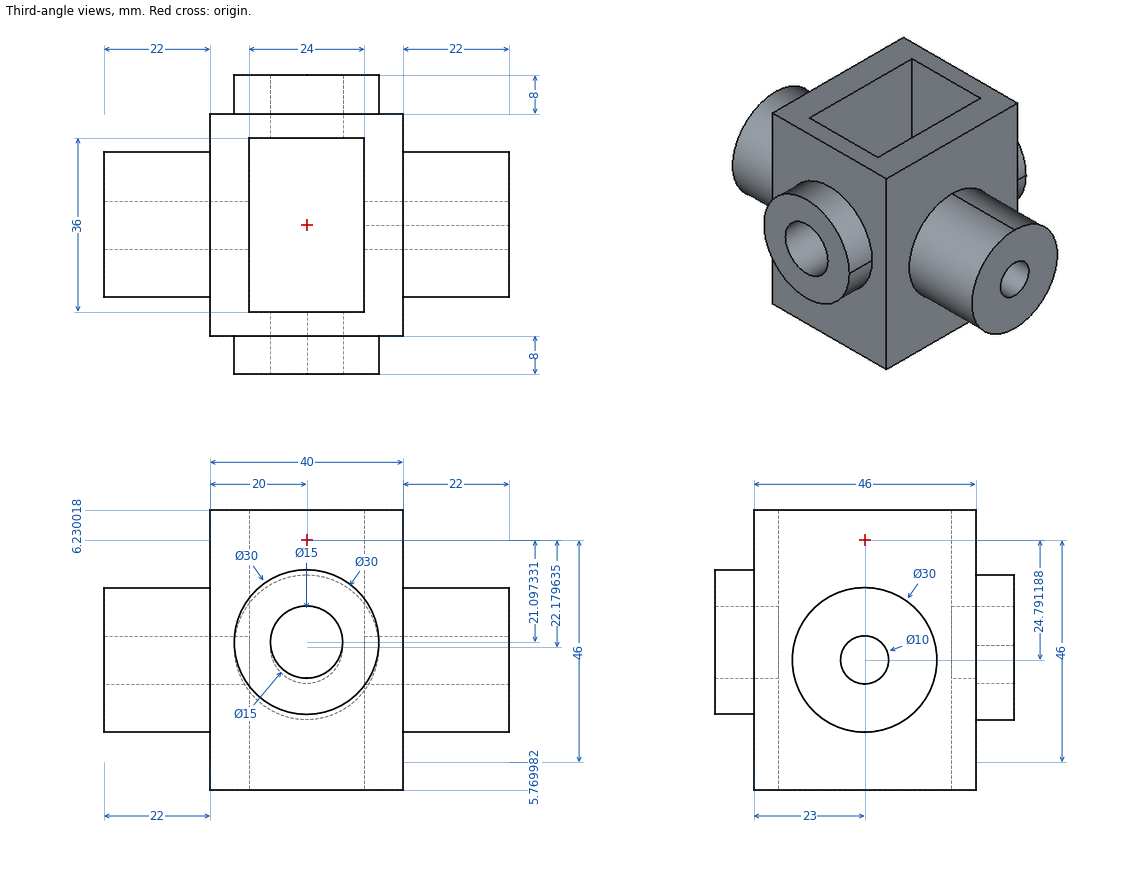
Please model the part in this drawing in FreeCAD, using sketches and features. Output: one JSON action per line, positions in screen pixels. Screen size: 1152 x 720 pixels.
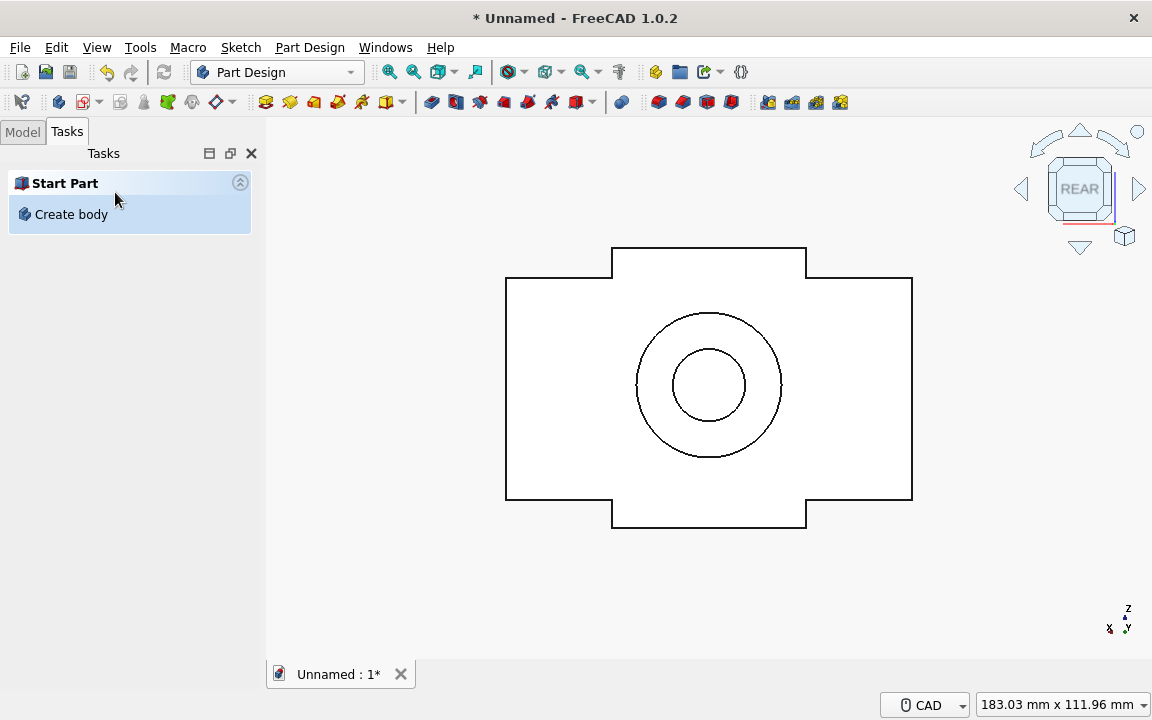
{"action": "key", "text": "0"}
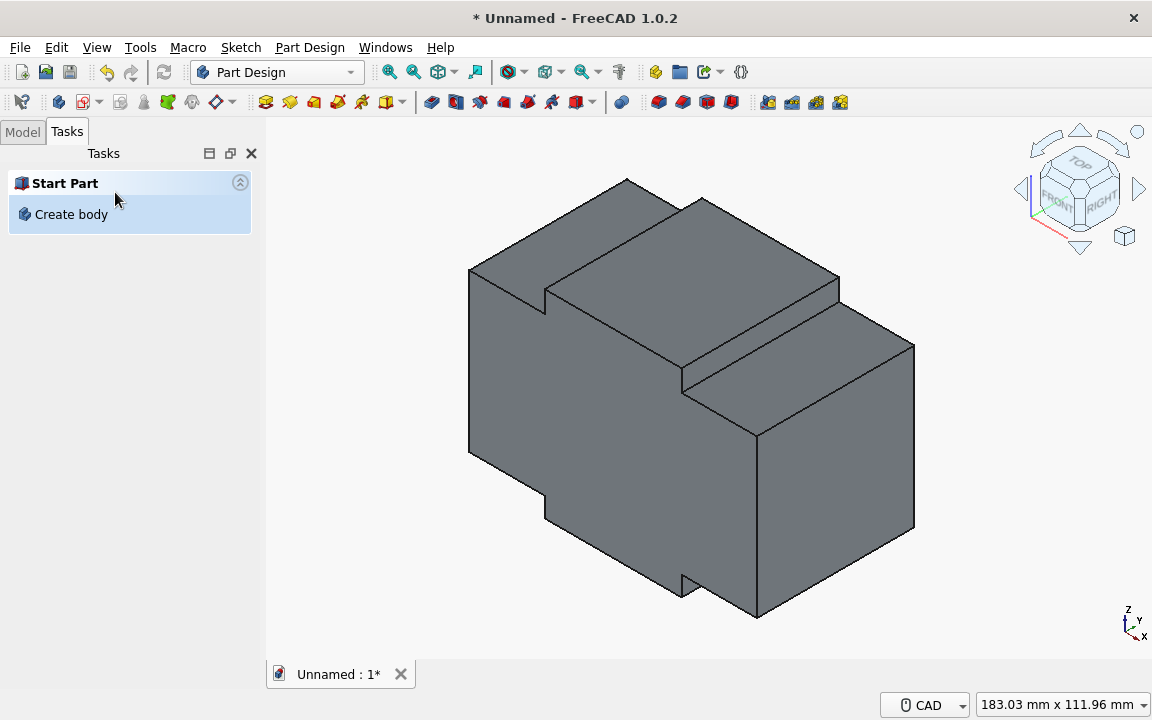
{"action": "left_click", "coordinate": [692, 282]}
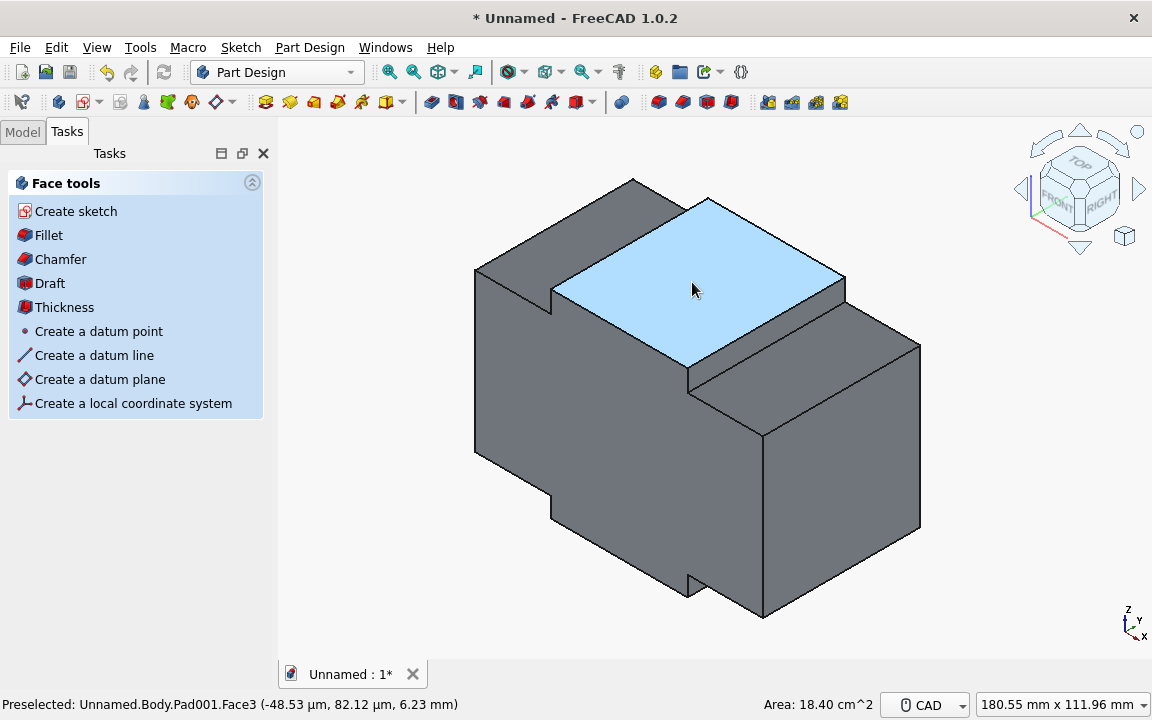
{"action": "left_click", "coordinate": [84, 102]}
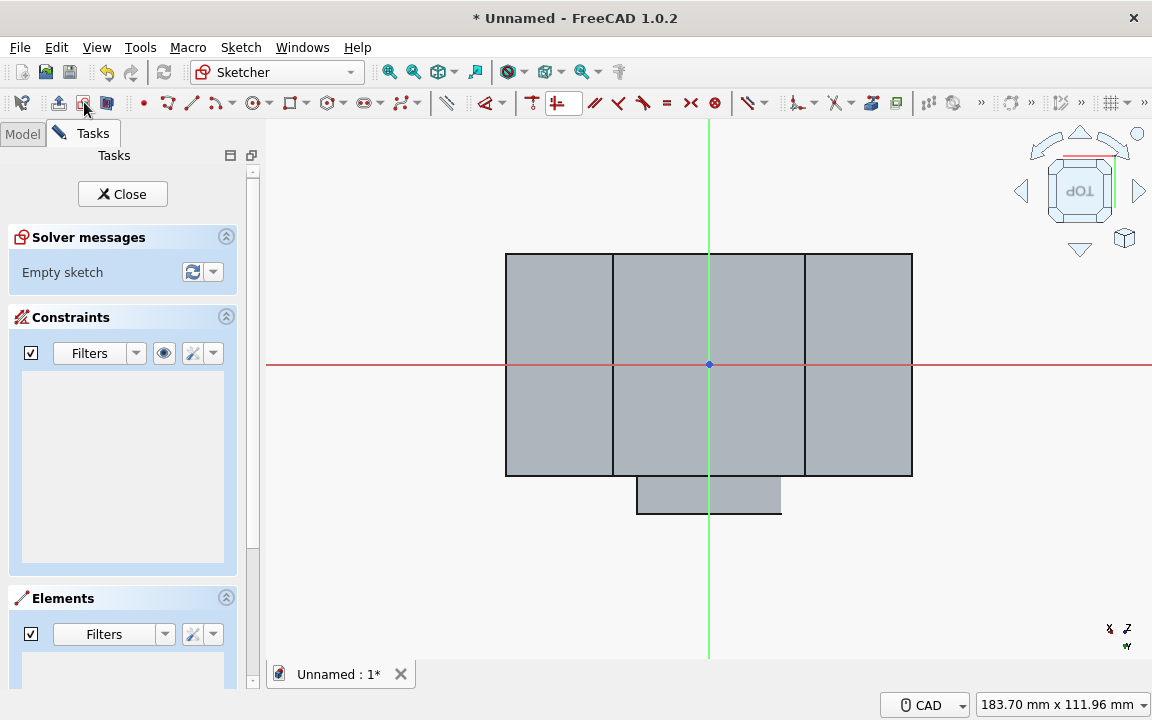
{"action": "scroll", "coordinate": [792, 336], "scroll_direction": "up", "scroll_amount": 3}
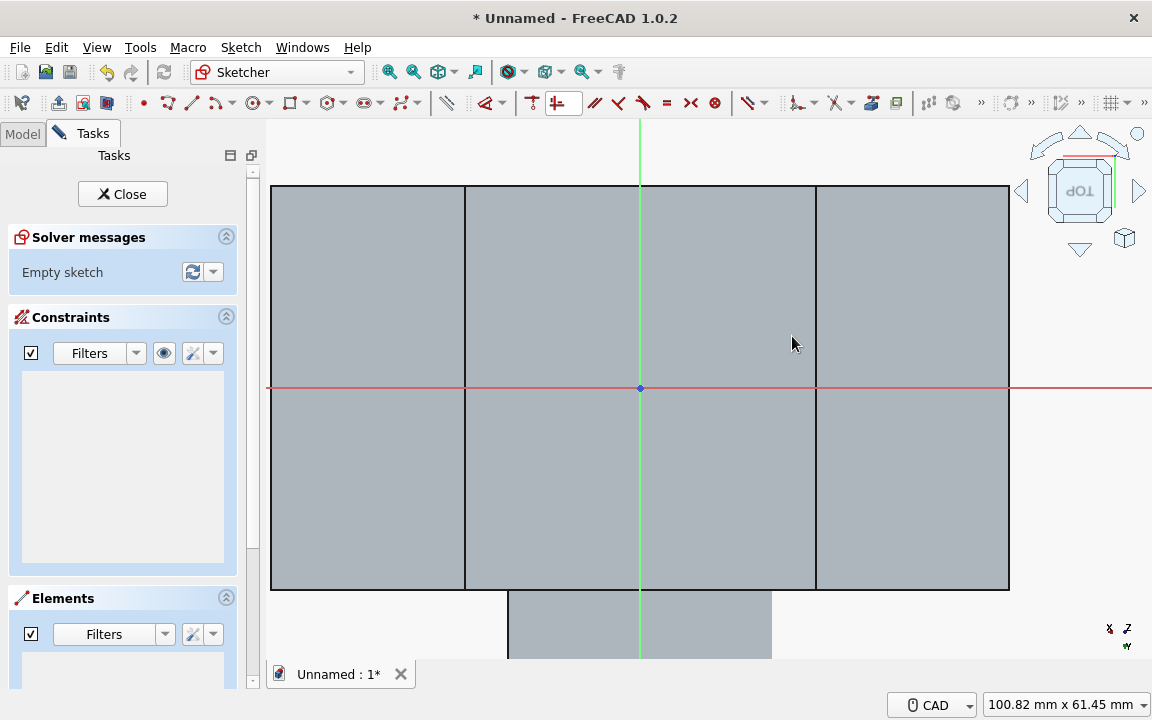
{"action": "key", "text": "g v"}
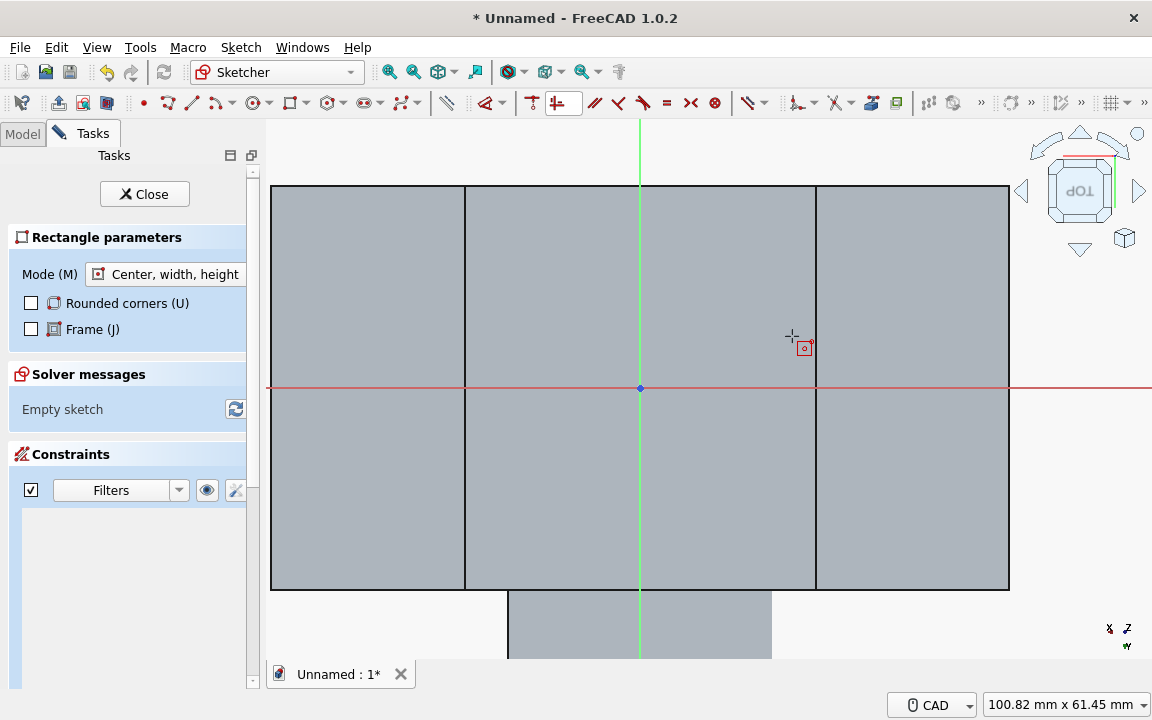
{"action": "left_click", "coordinate": [640, 388]}
{"action": "left_click", "coordinate": [746, 230]}
{"action": "key", "text": "Escape"}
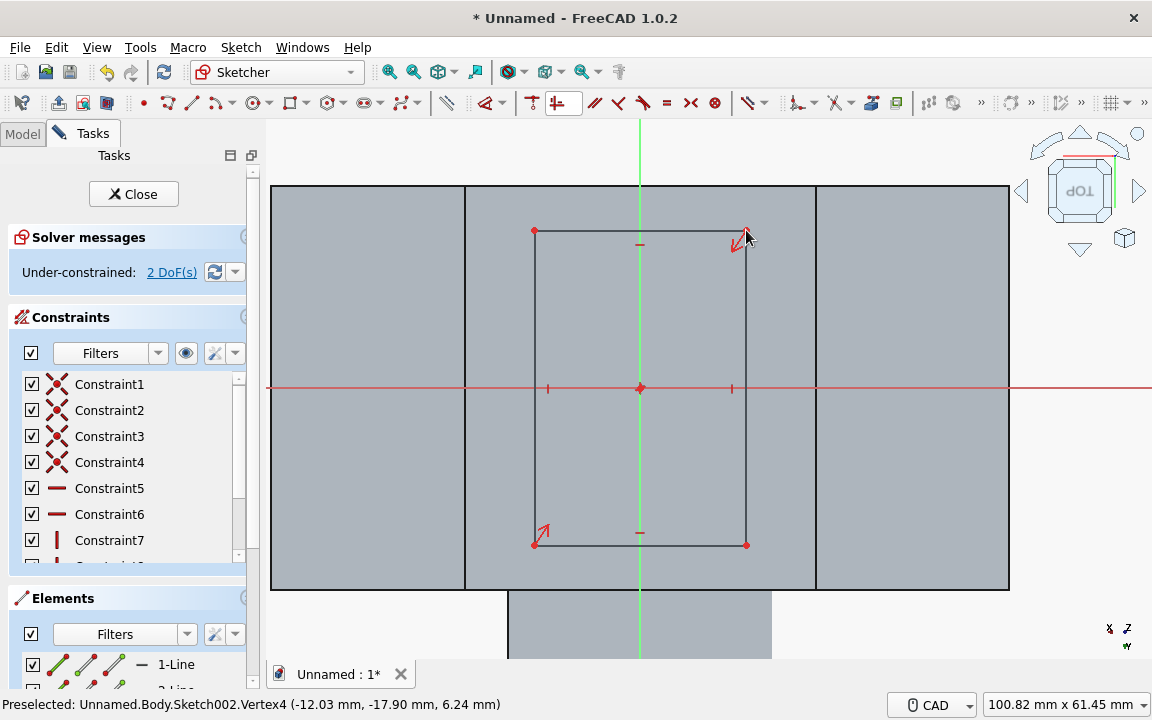
{"action": "left_click", "coordinate": [486, 104]}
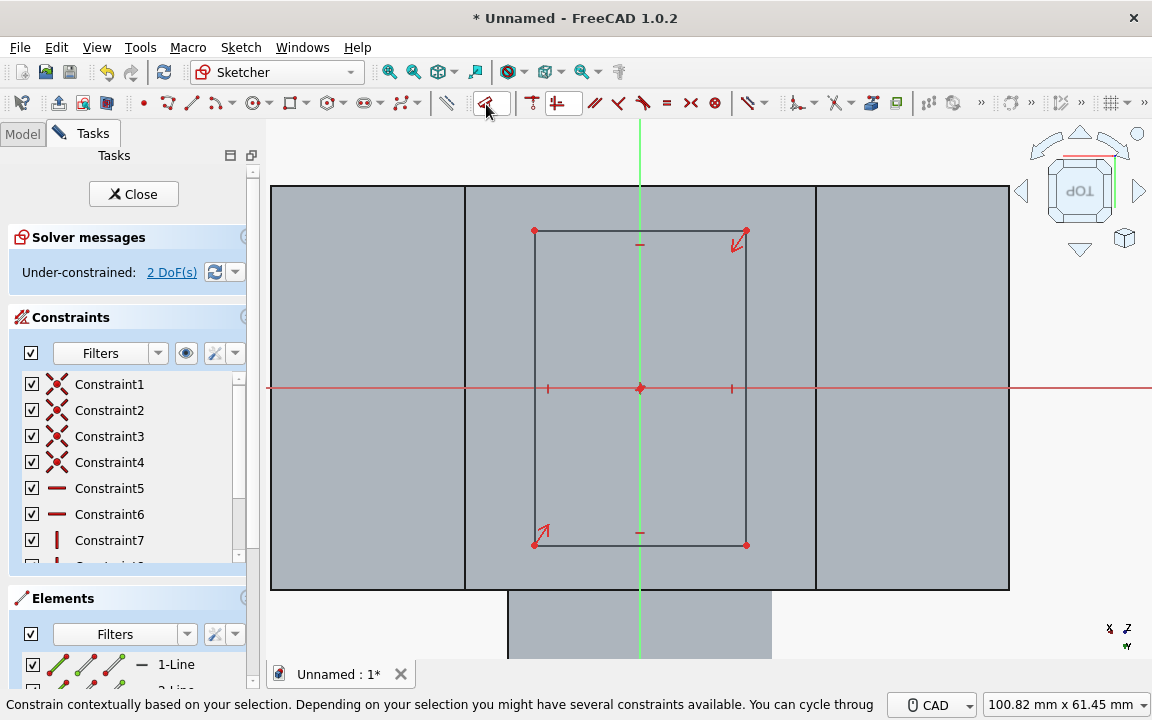
{"action": "left_click", "coordinate": [598, 546]}
{"action": "left_click", "coordinate": [592, 580]}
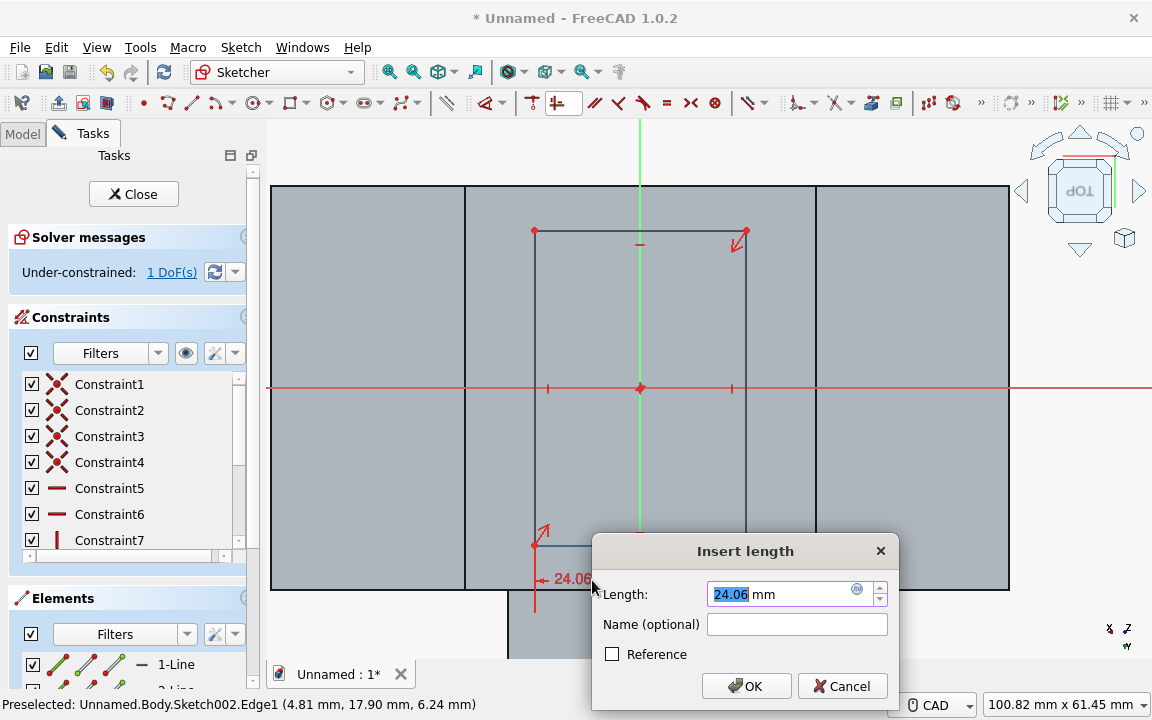
{"action": "type", "text": "24"}
{"action": "key", "text": "Return"}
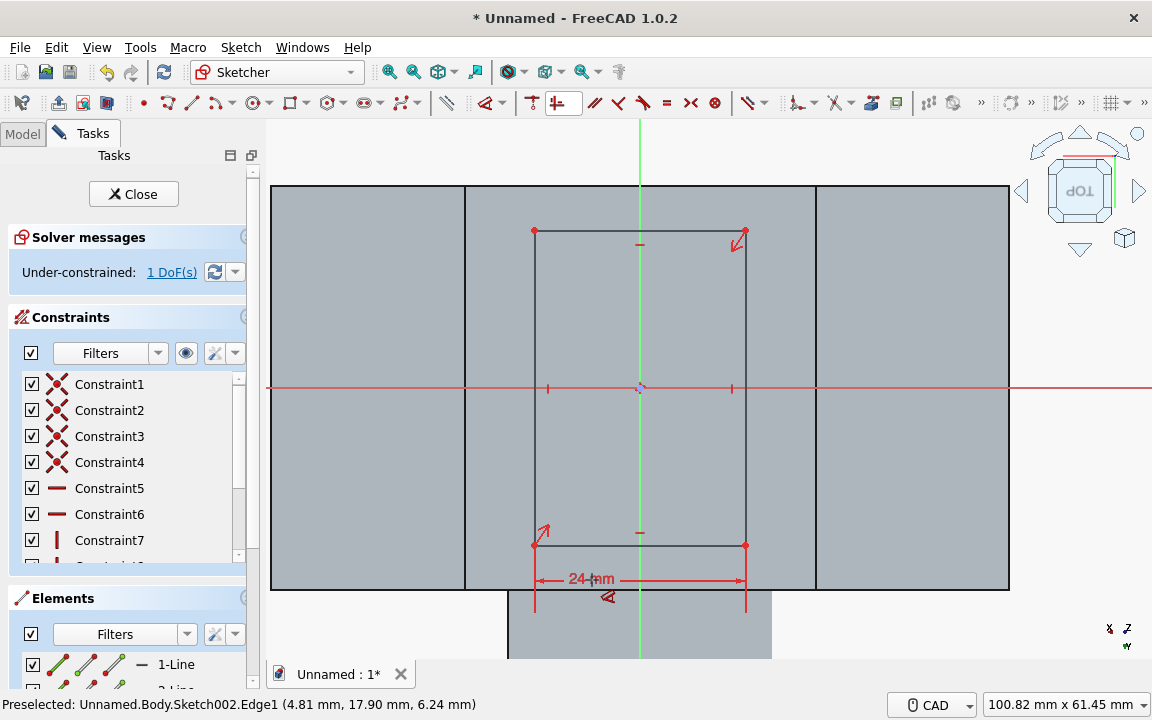
{"action": "left_click", "coordinate": [746, 451]}
{"action": "left_click", "coordinate": [780, 316]}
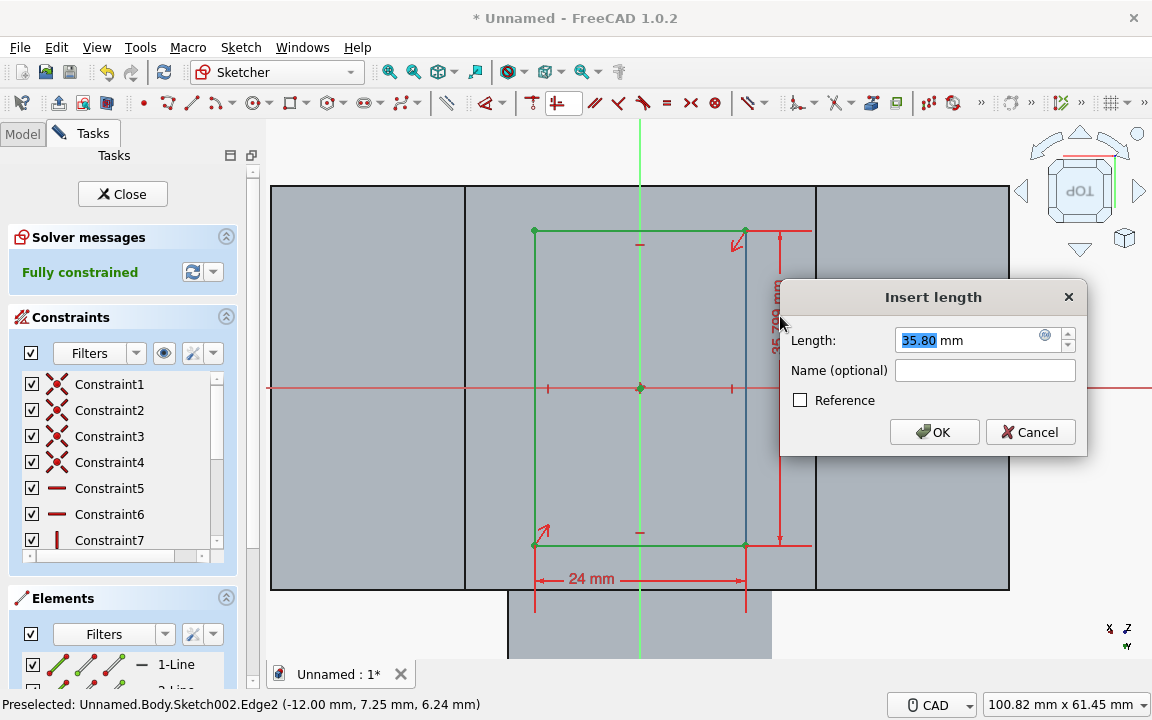
{"action": "type", "text": "36"}
{"action": "key", "text": "Return"}
{"action": "key", "text": "Escape"}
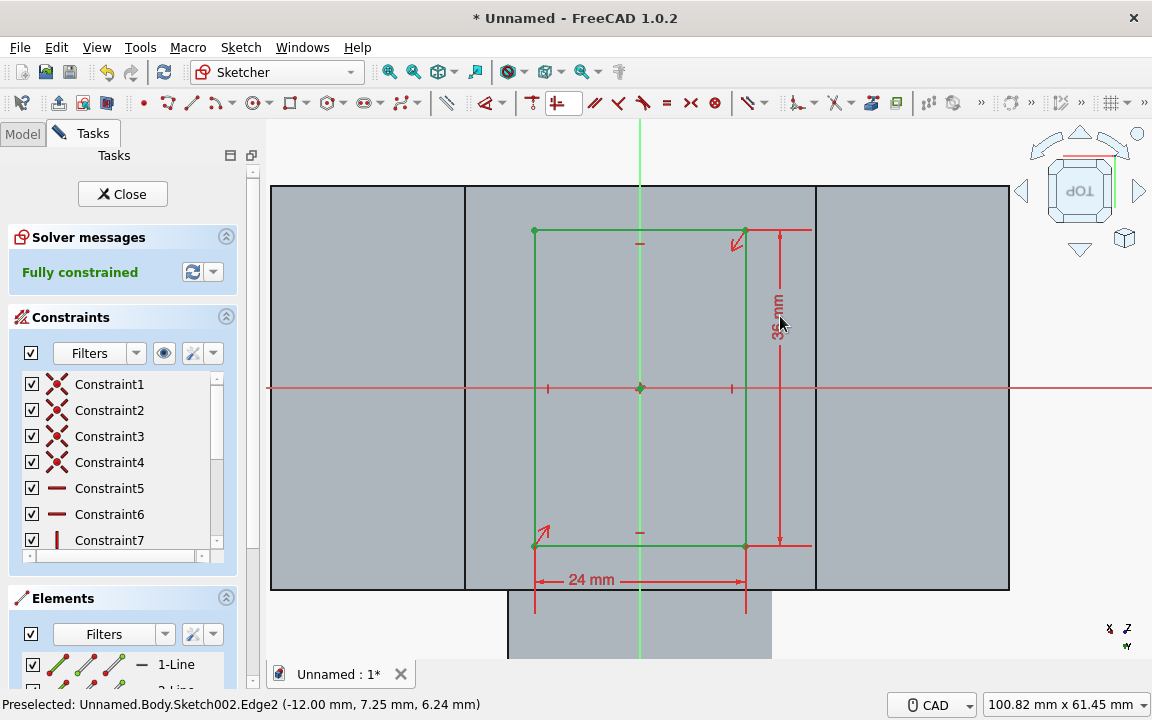
{"action": "left_click", "coordinate": [123, 194]}